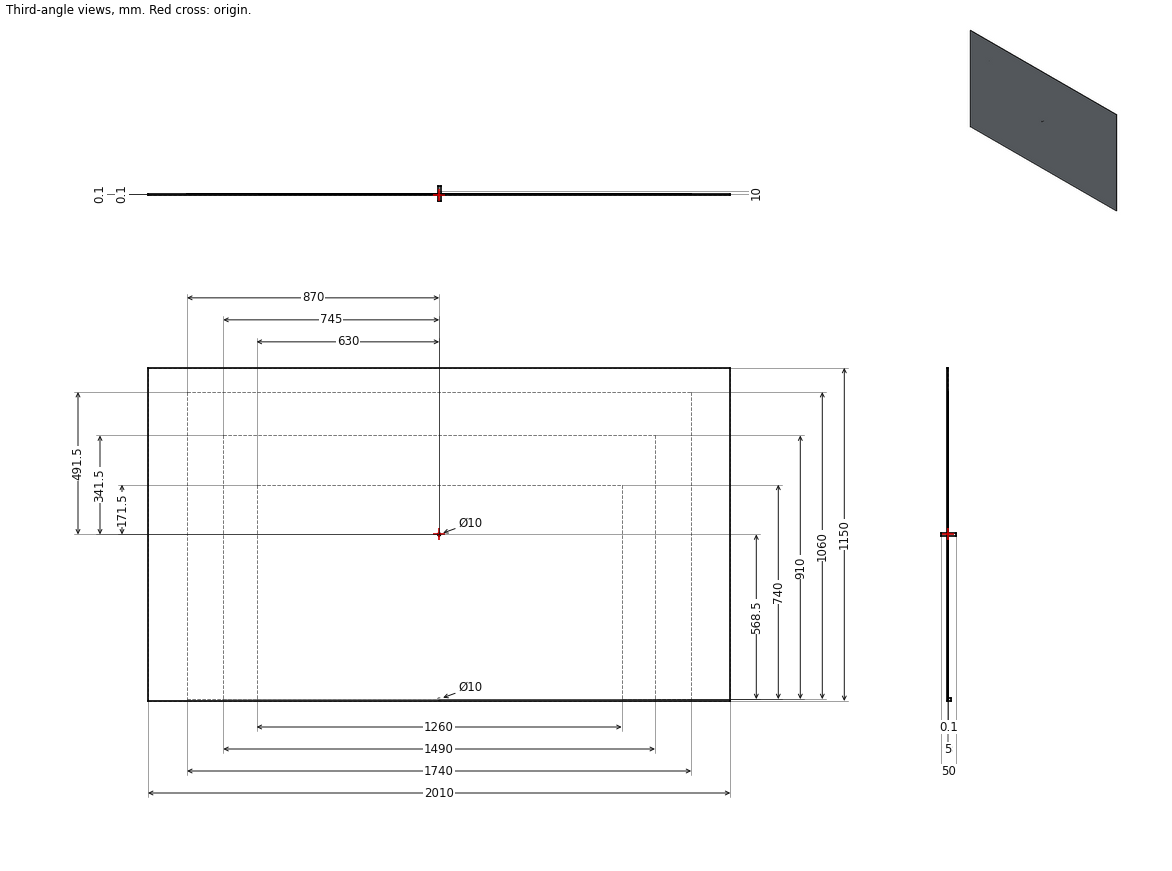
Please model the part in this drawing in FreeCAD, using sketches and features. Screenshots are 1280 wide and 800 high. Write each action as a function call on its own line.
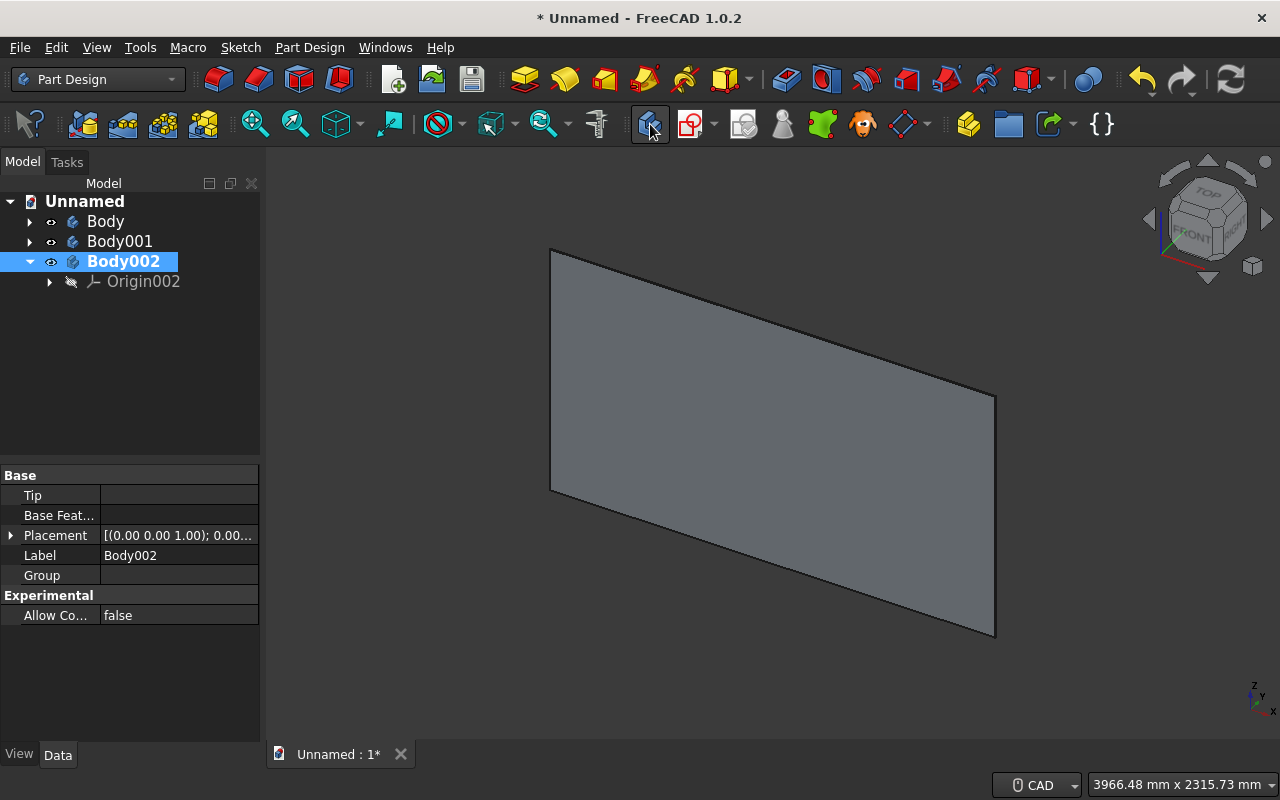
click(50, 282)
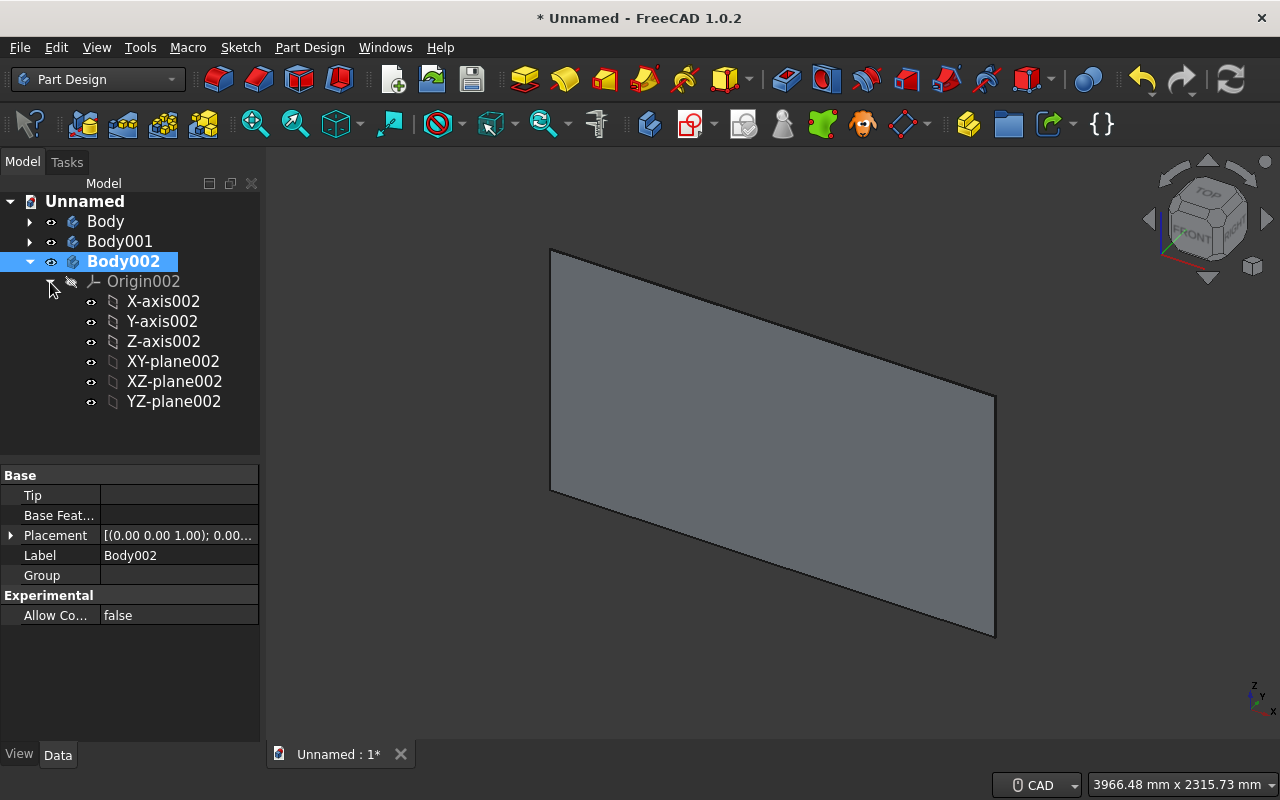
click(136, 382)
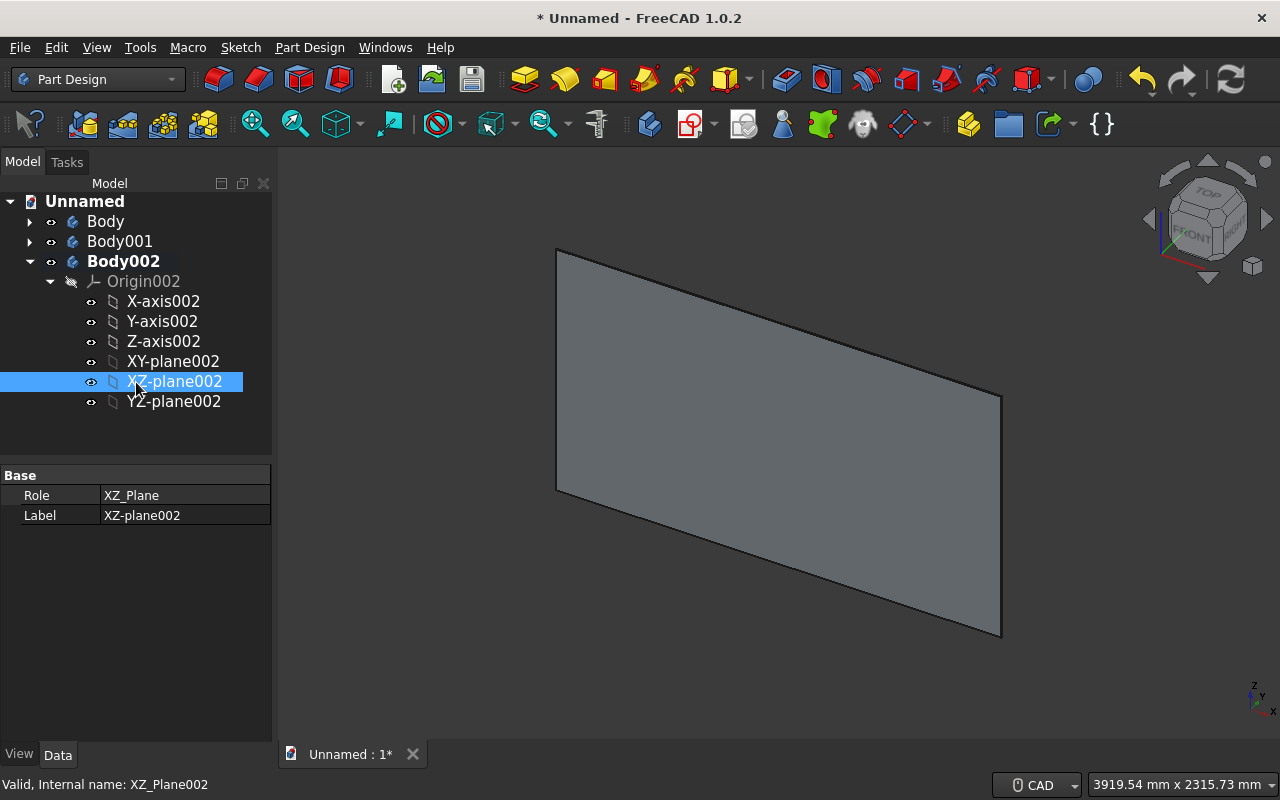
click(904, 124)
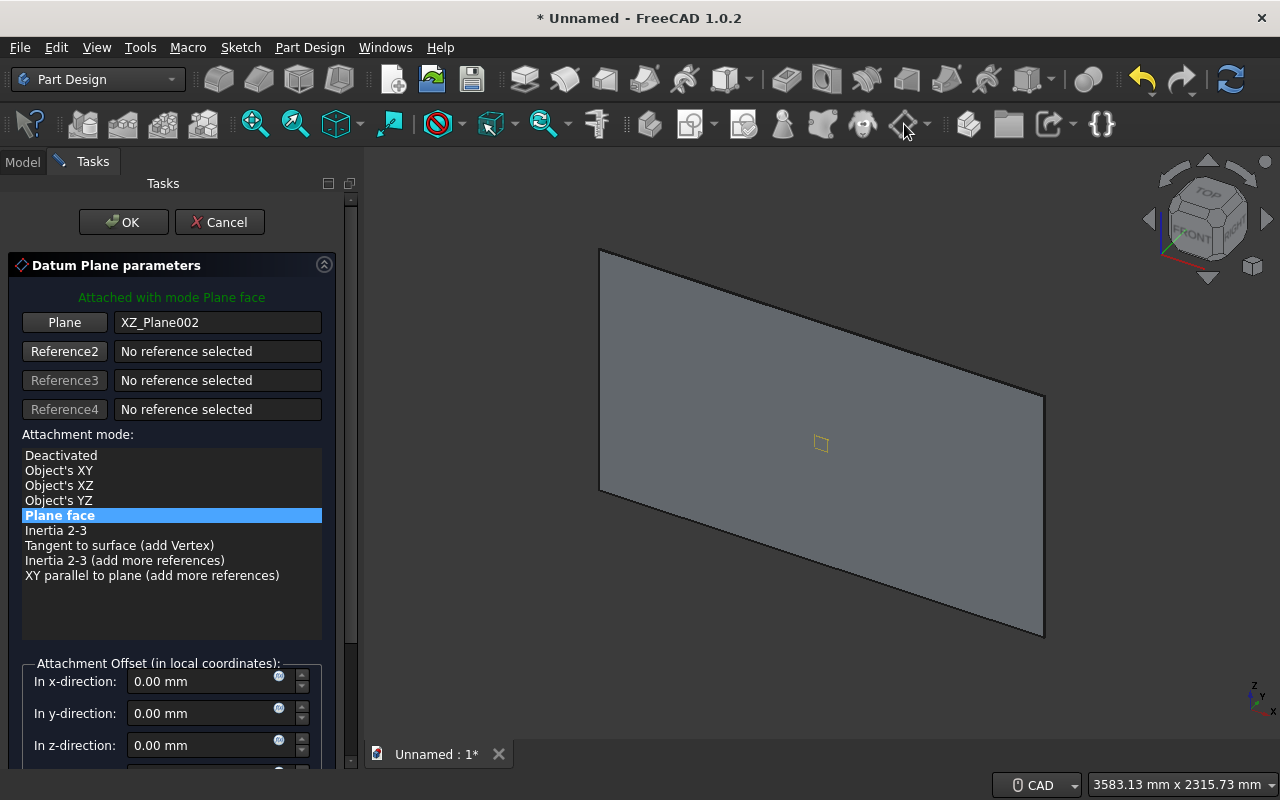
triple_click(210, 745)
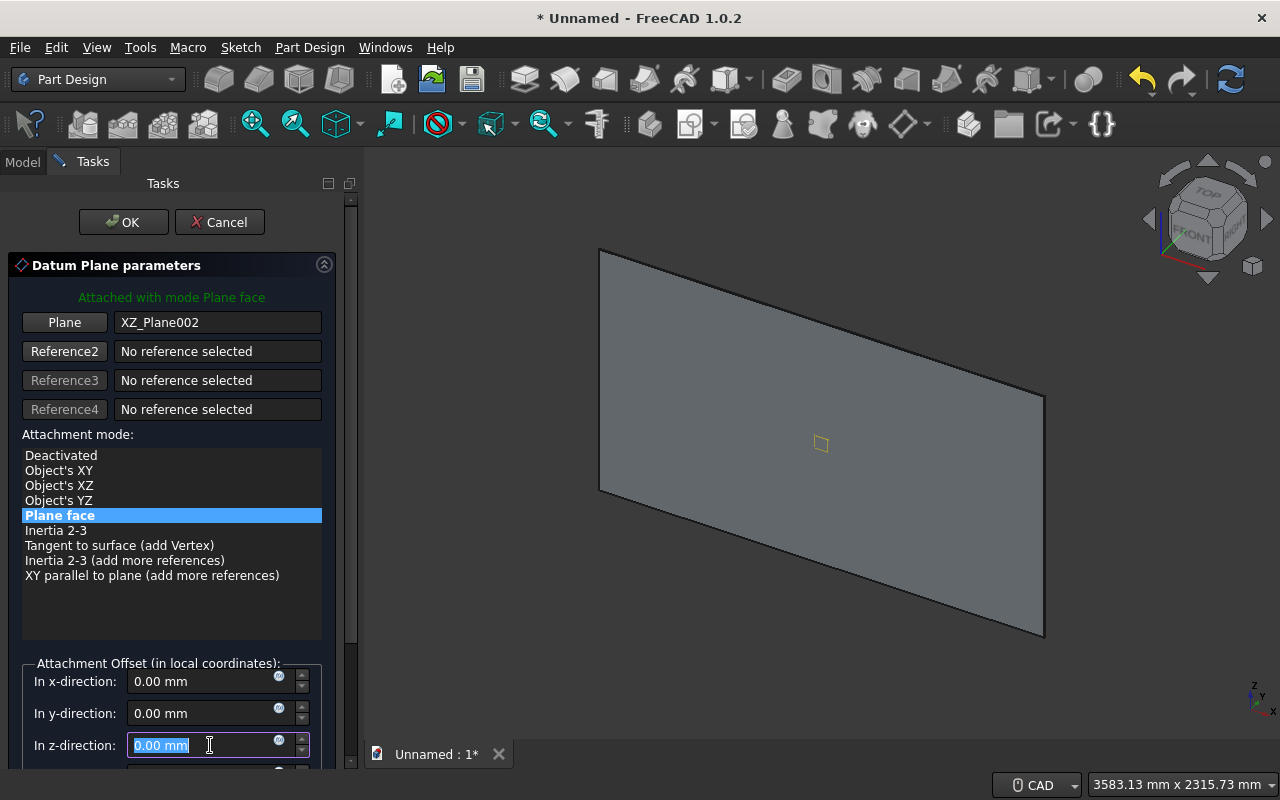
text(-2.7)
key(Tab)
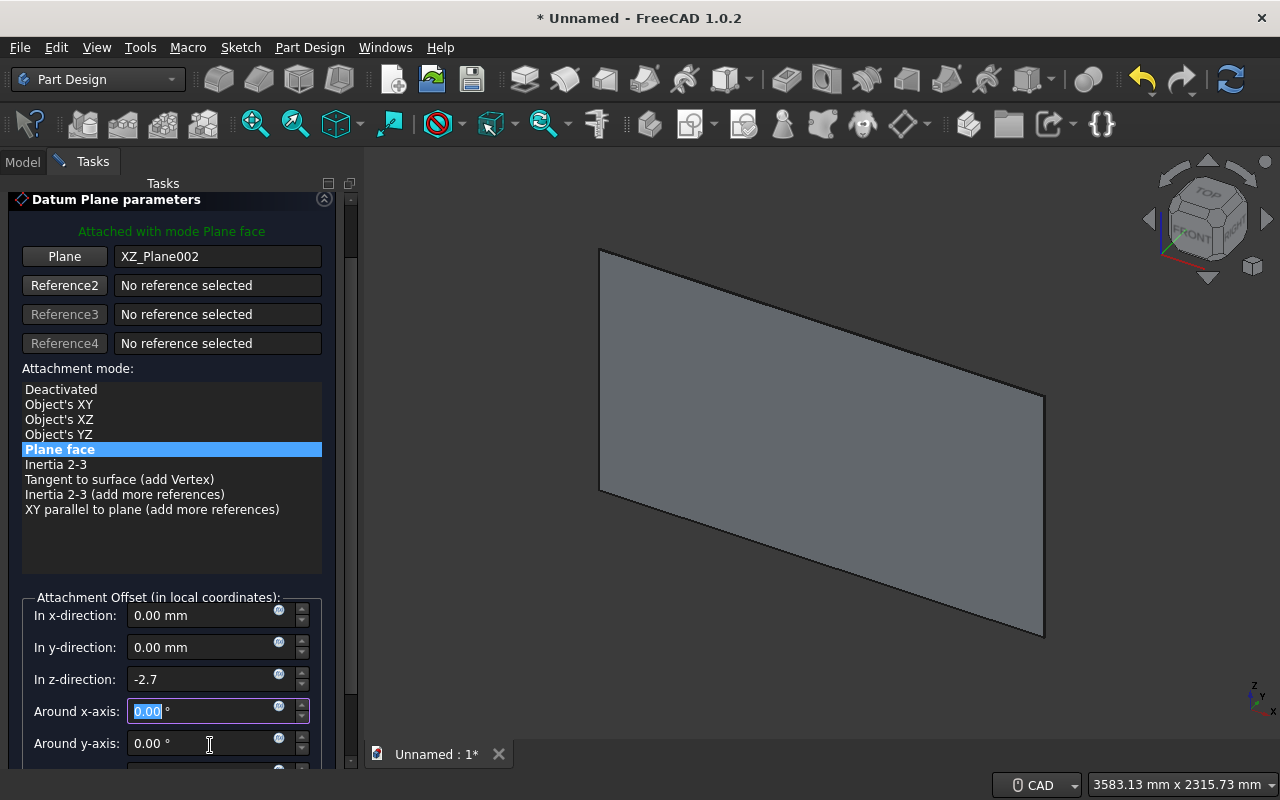
scroll(351, 480, up, 2)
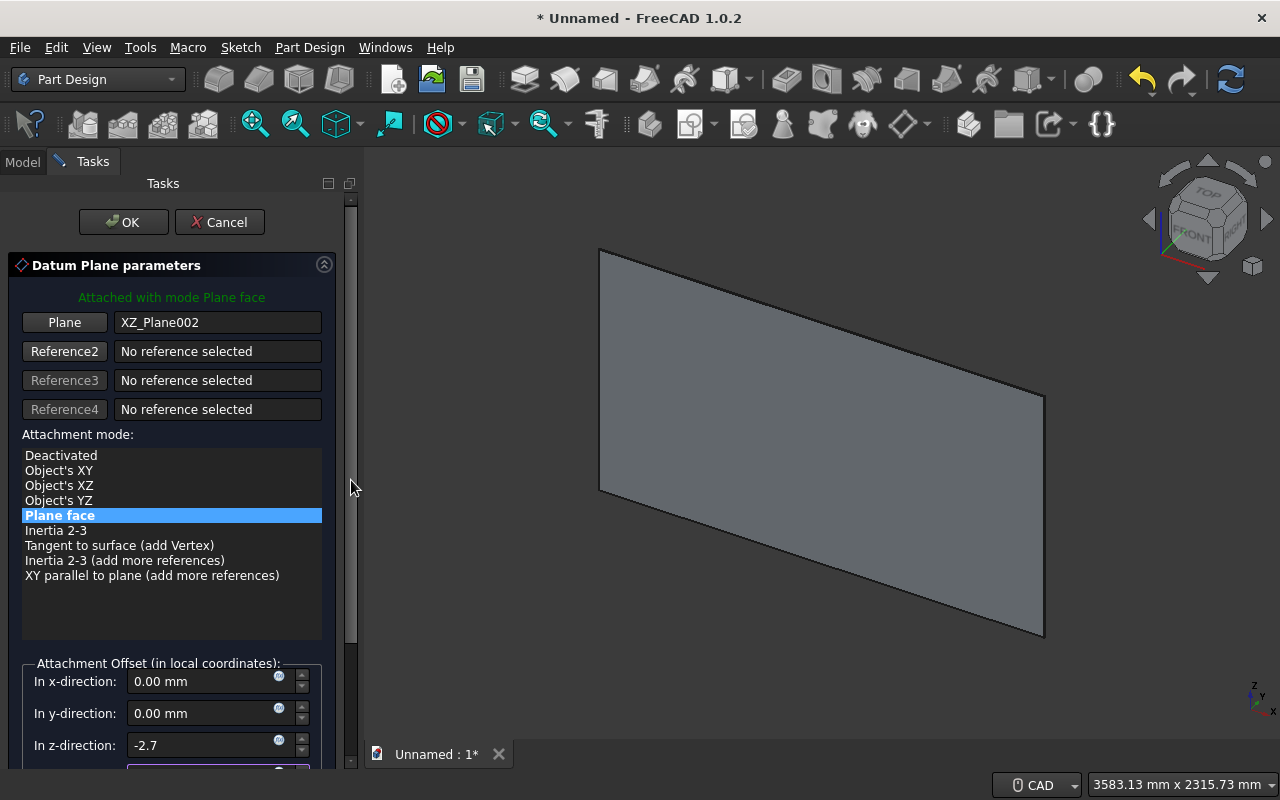
click(124, 222)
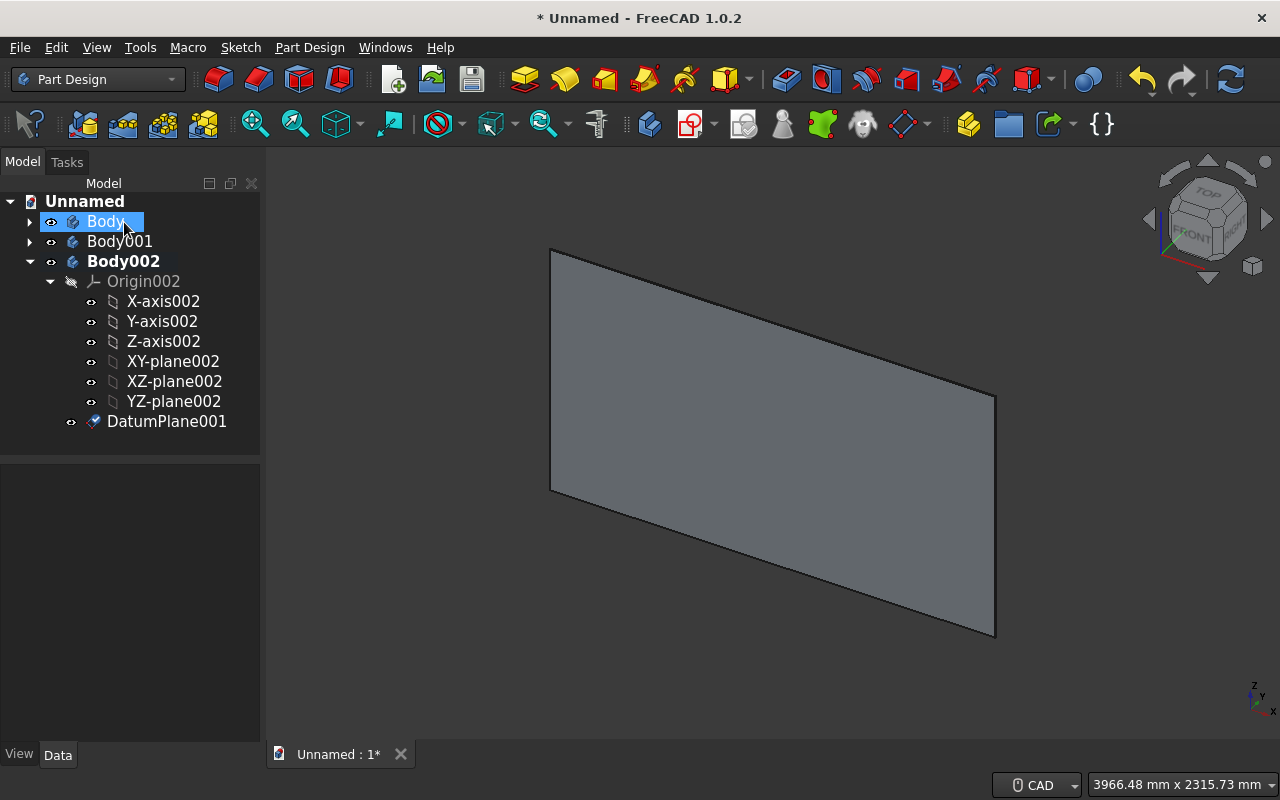
click(116, 422)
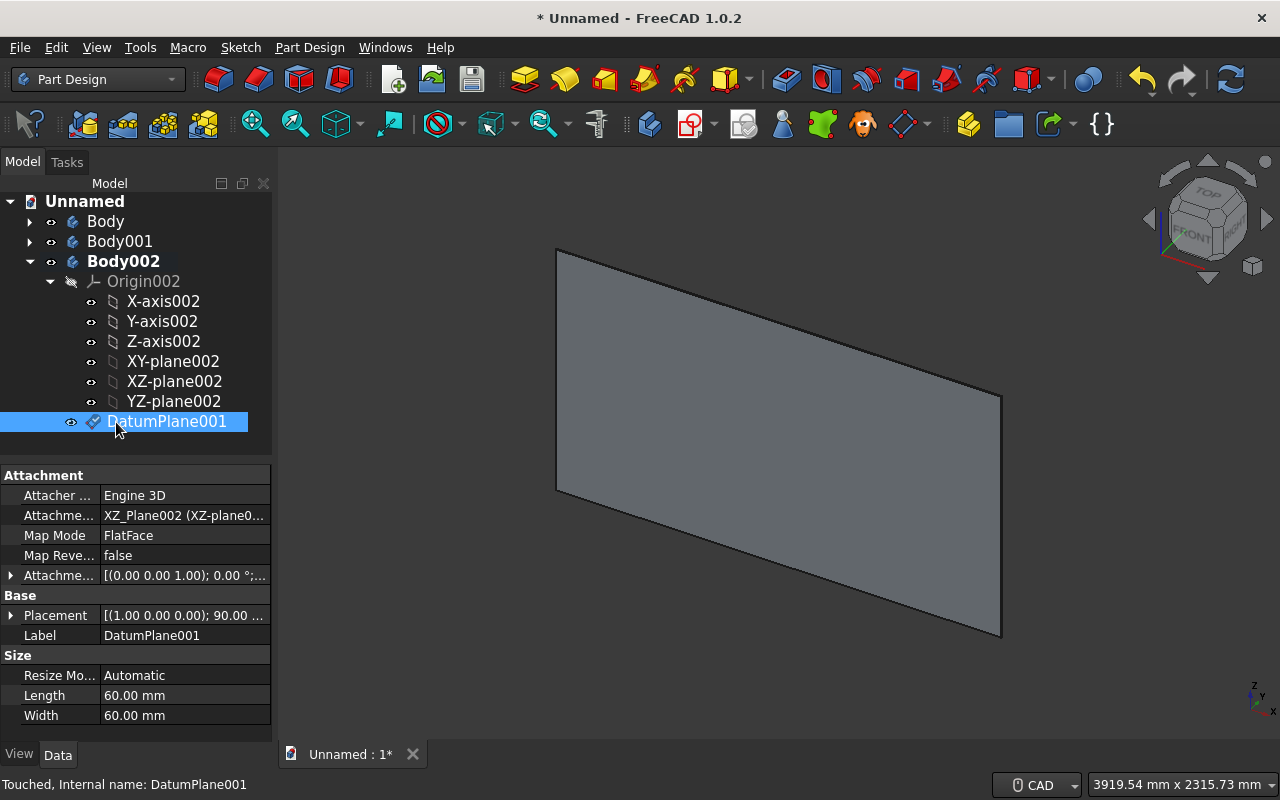
click(690, 124)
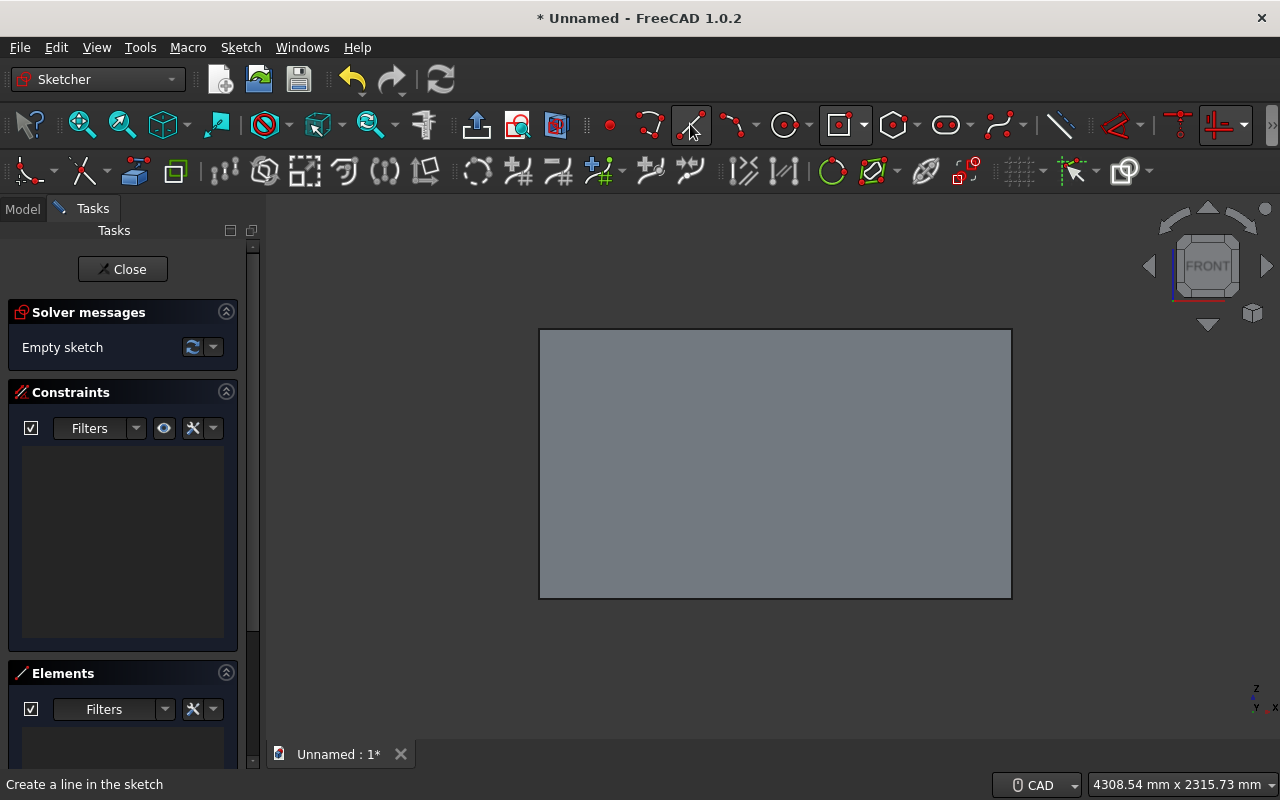
scroll(919, 539, up, 2)